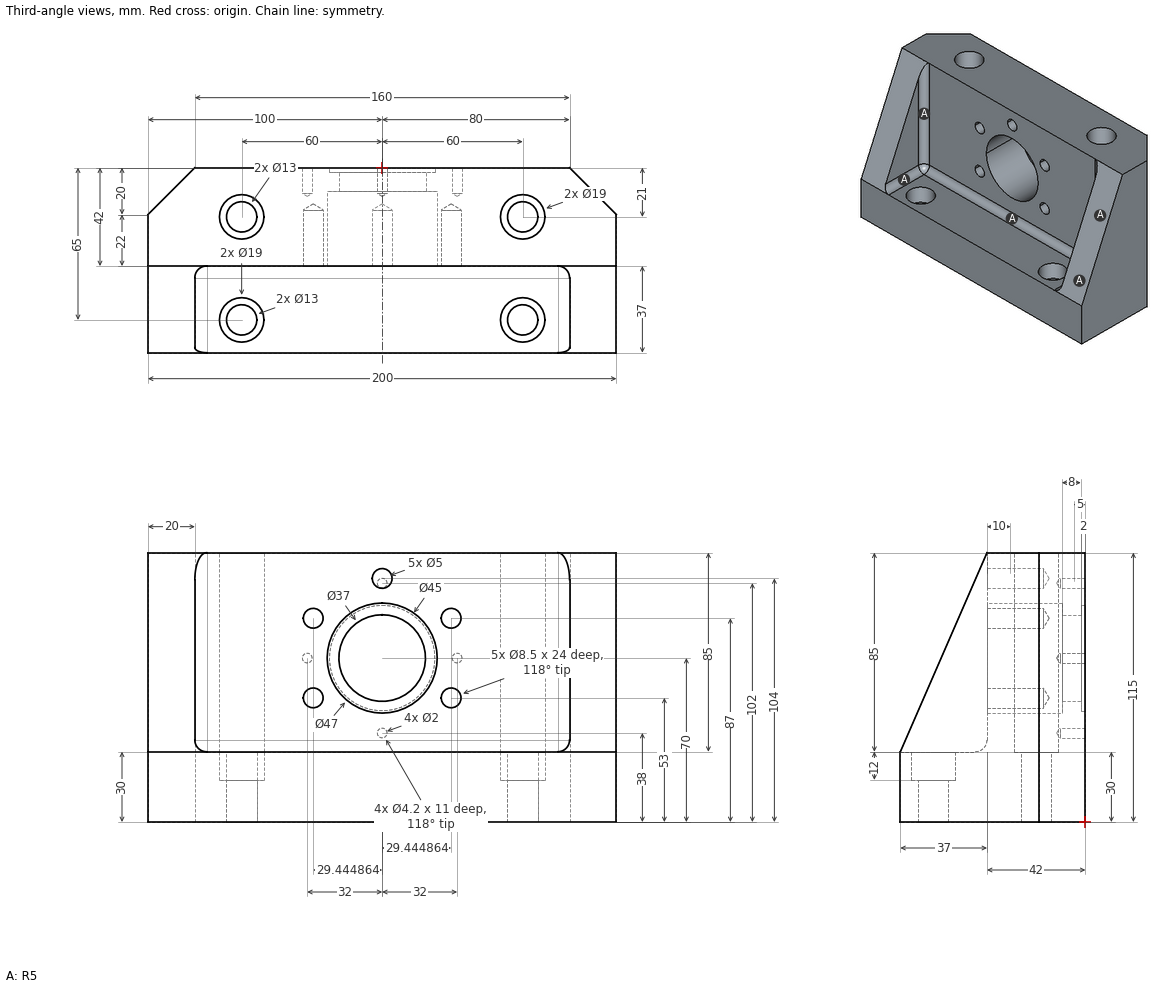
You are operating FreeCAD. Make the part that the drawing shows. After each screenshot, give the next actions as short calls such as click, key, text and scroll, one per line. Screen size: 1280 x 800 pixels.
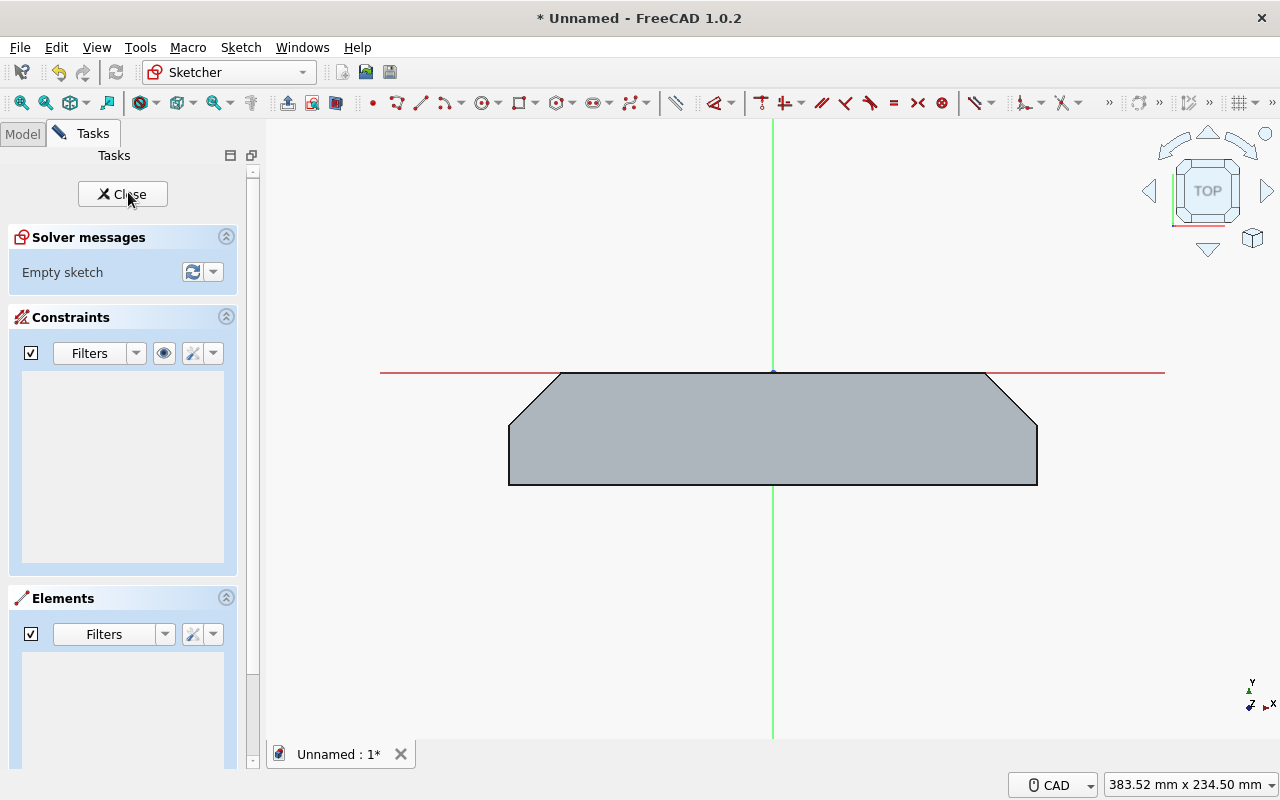
click(336, 104)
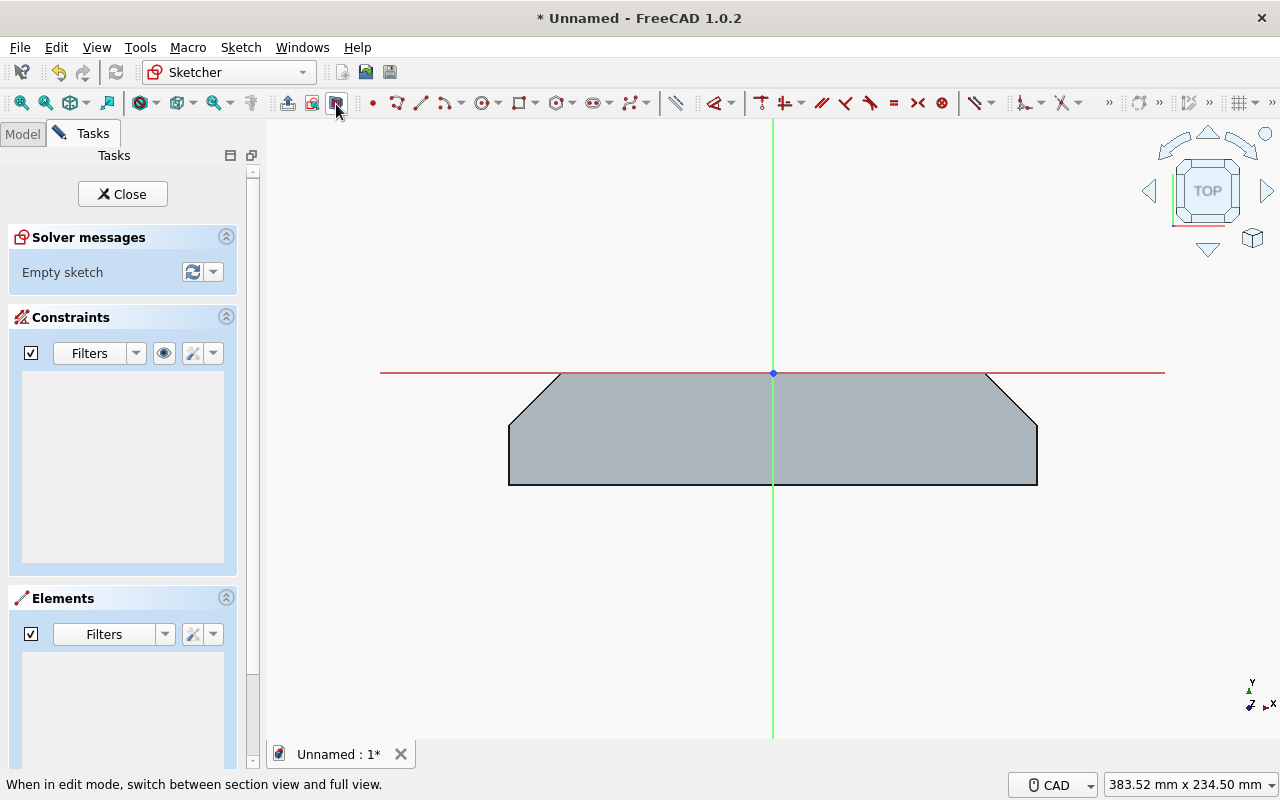
click(520, 104)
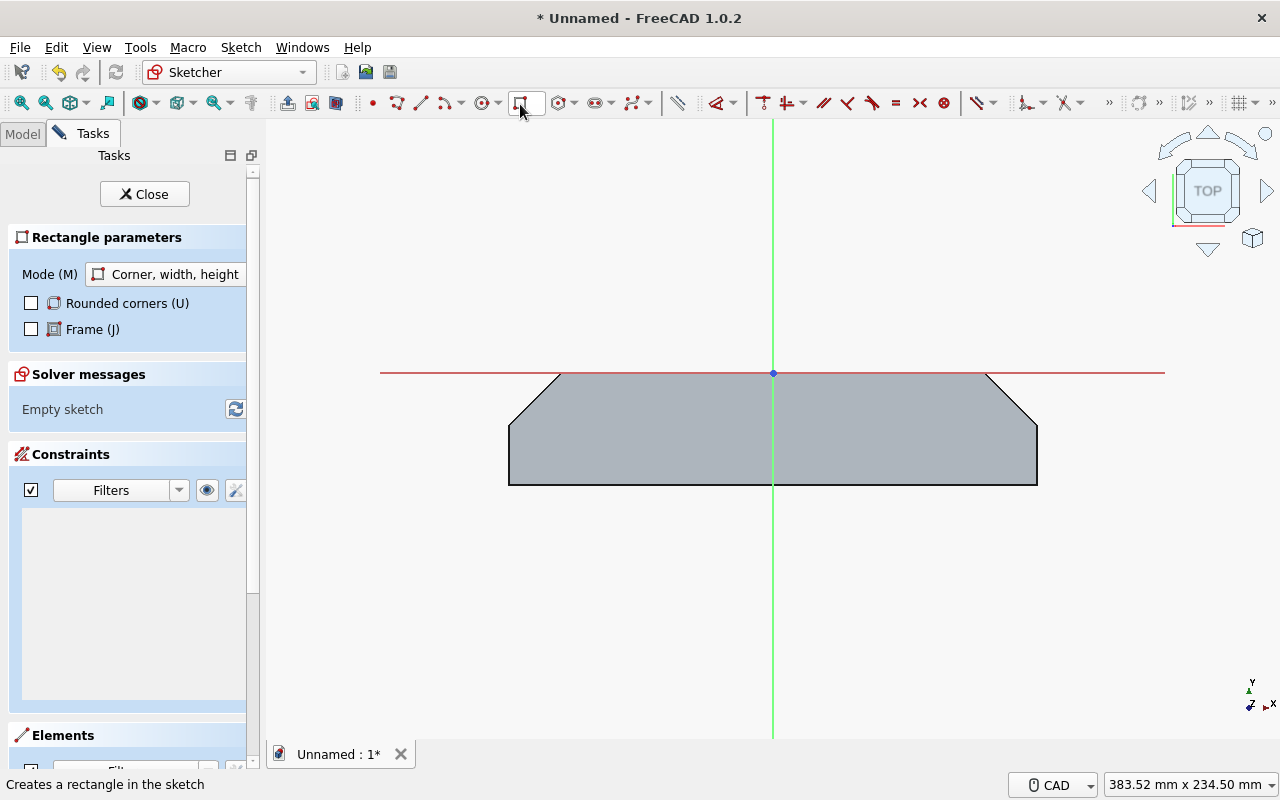
click(509, 485)
move(1037, 582)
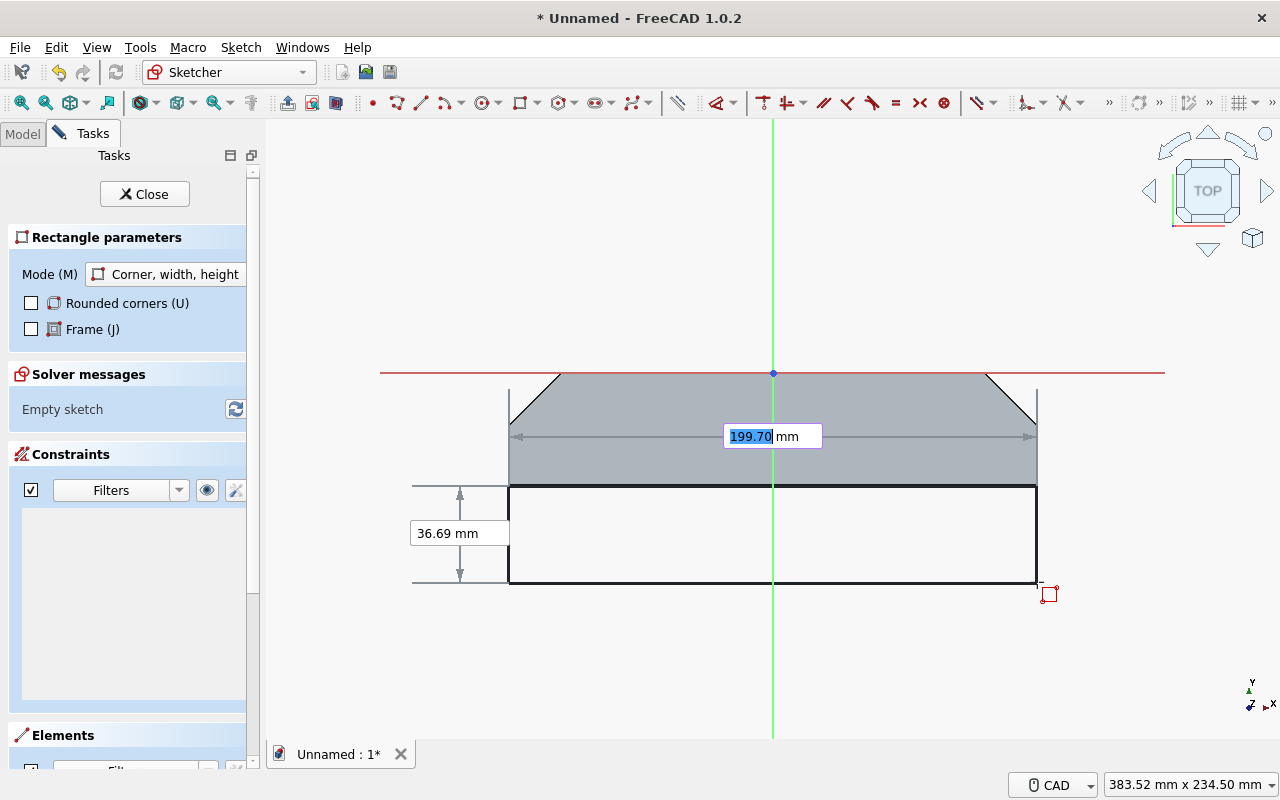
text(200)
key(Tab)
text(37)
key(Return)
key(Escape)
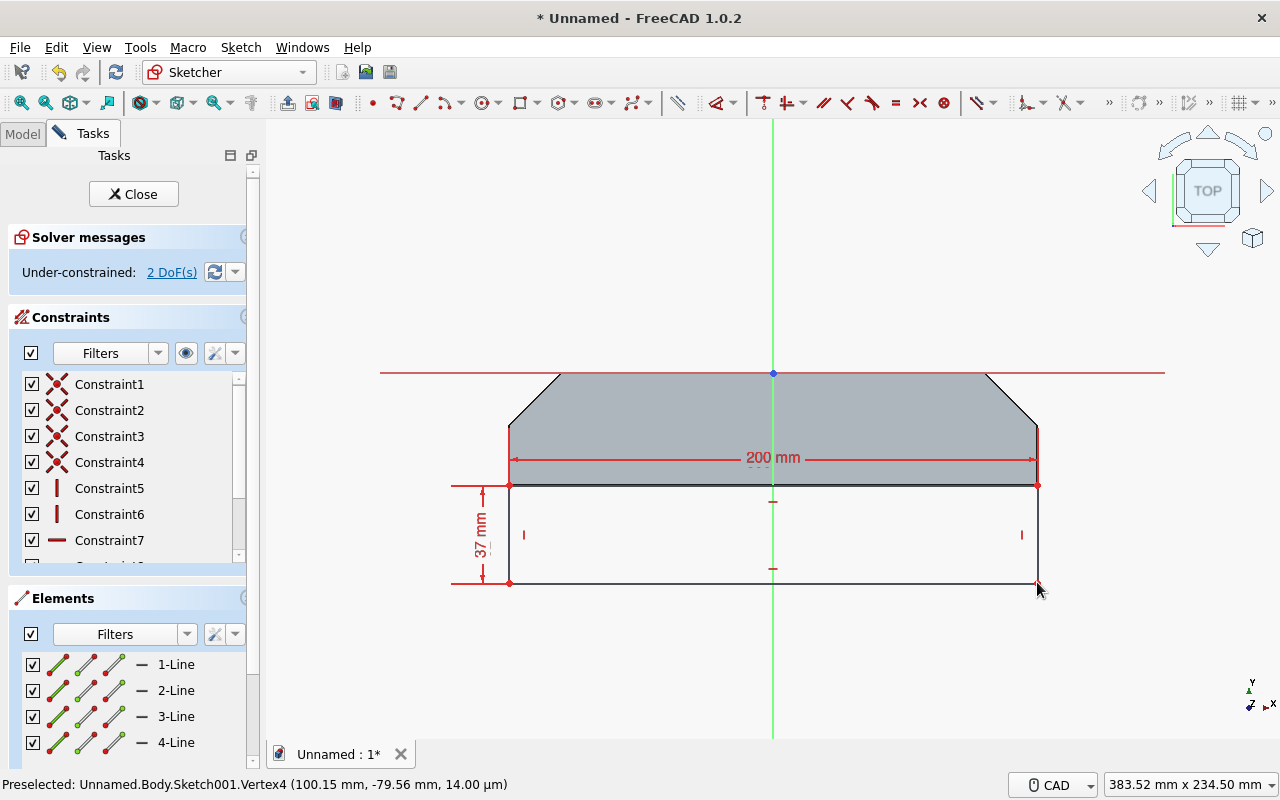
key(d)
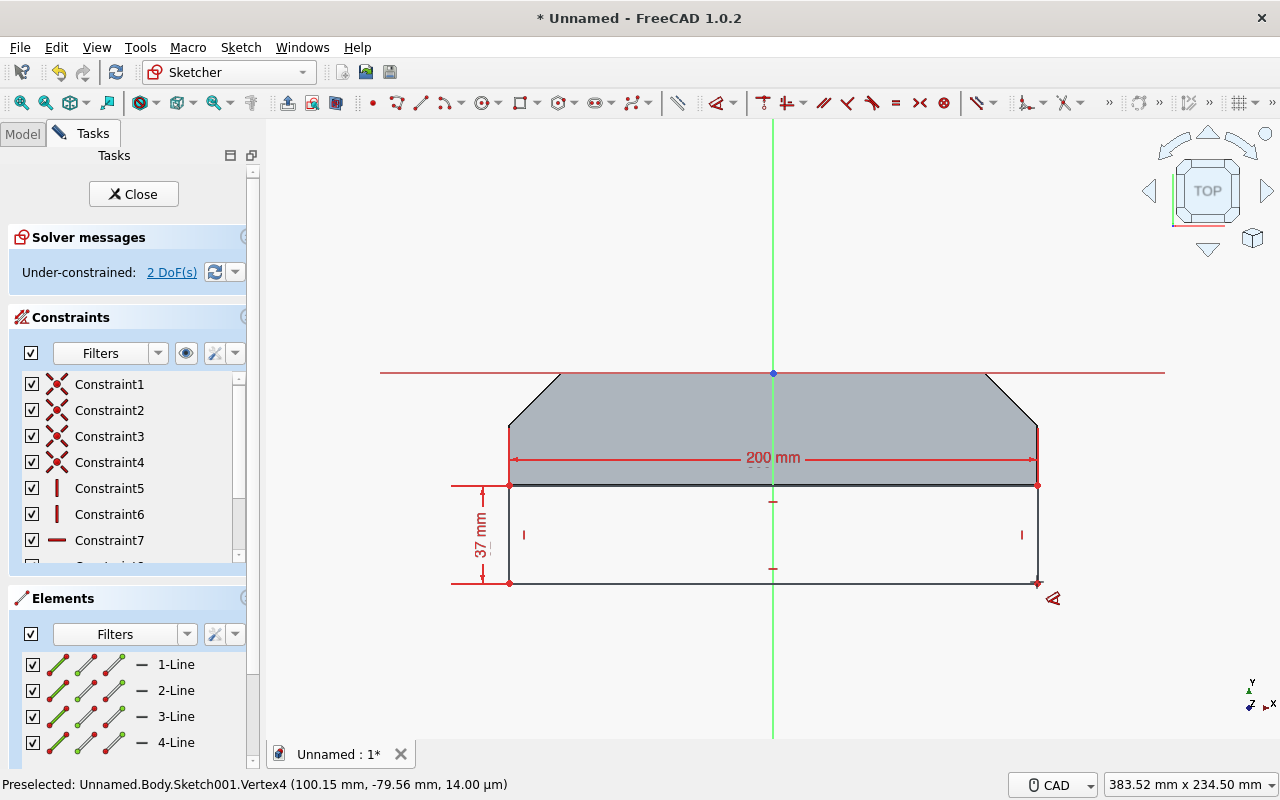
click(509, 486)
click(475, 430)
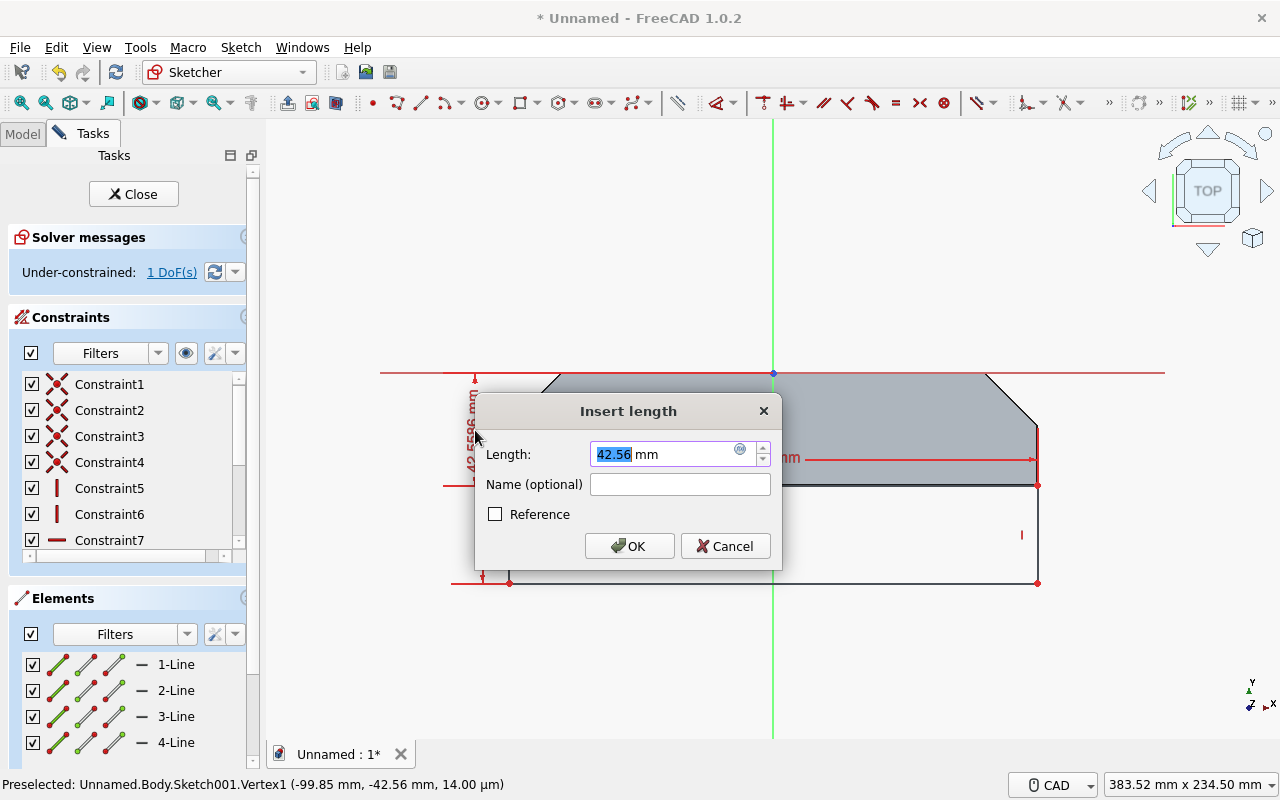
text(42)
key(Return)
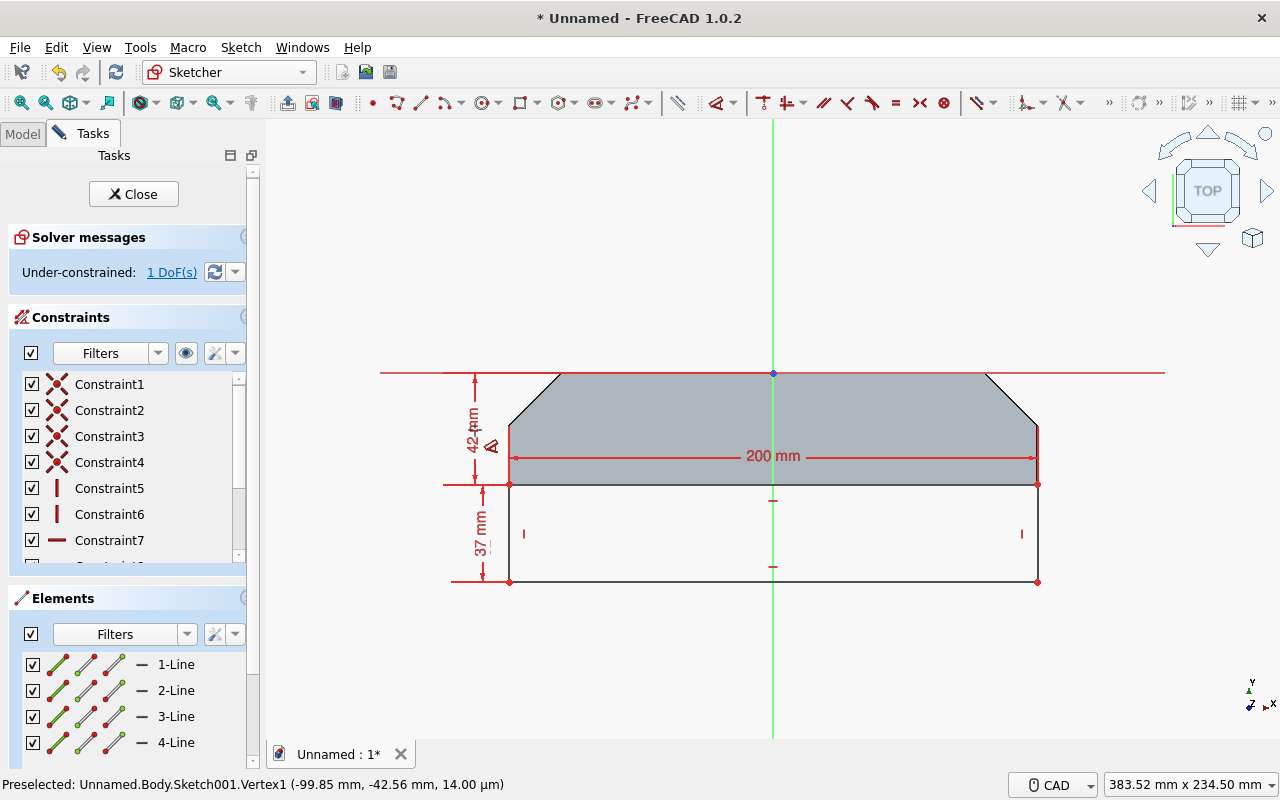
click(509, 485)
click(641, 339)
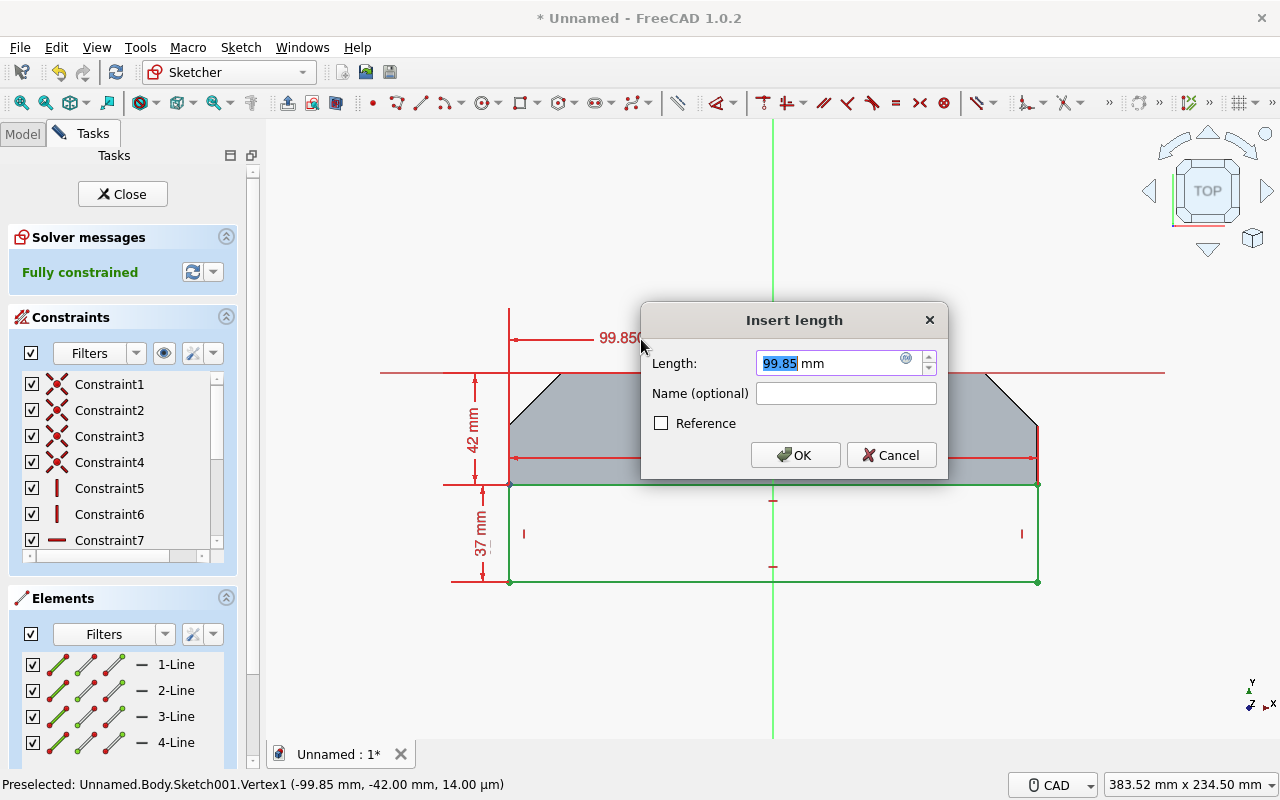
text(100)
key(Return)
key(Escape)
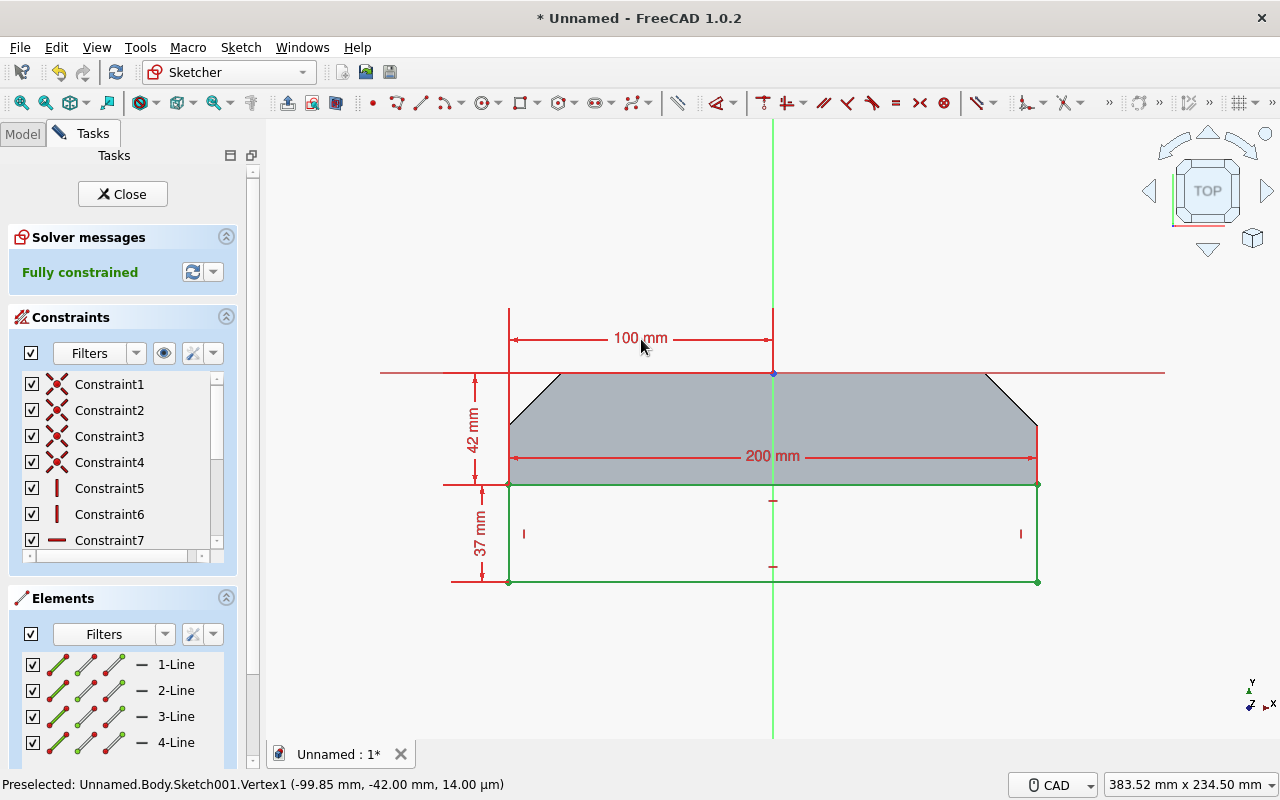
click(123, 194)